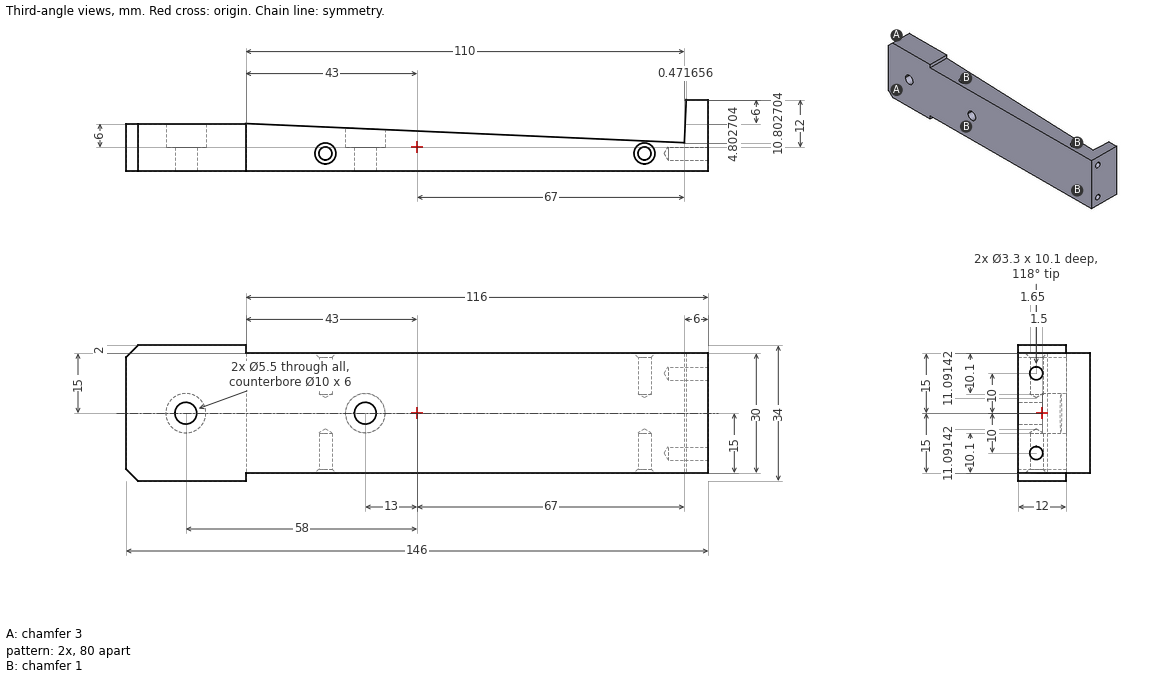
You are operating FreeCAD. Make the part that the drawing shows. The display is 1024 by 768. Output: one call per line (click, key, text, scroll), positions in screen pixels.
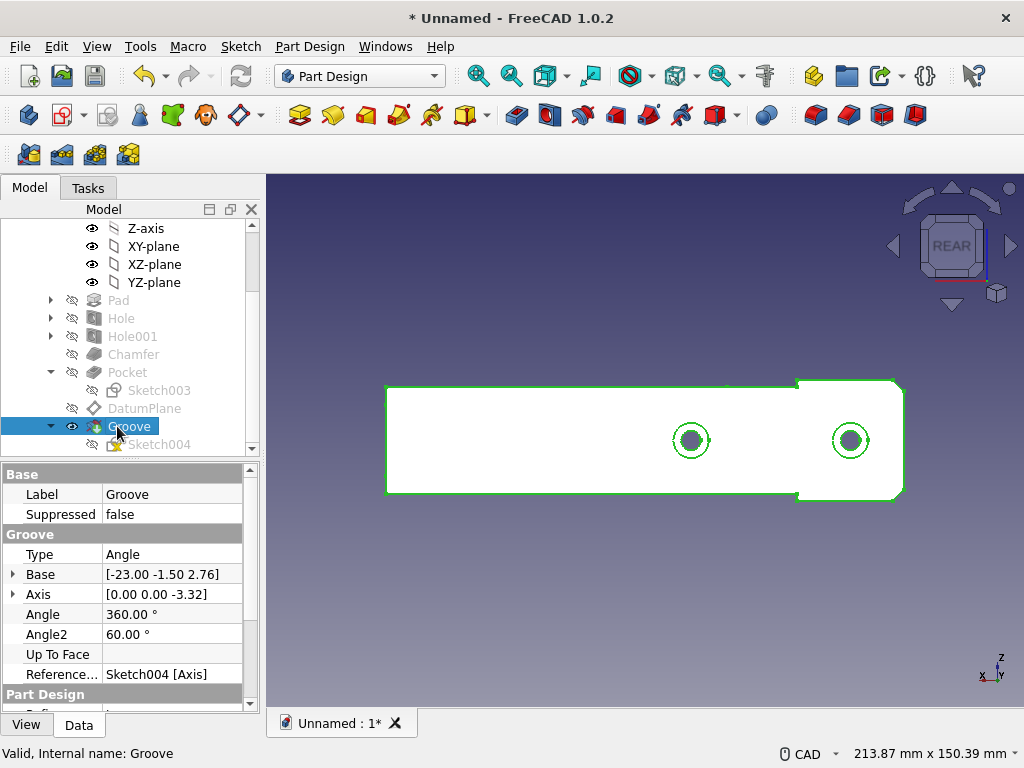
click(62, 154)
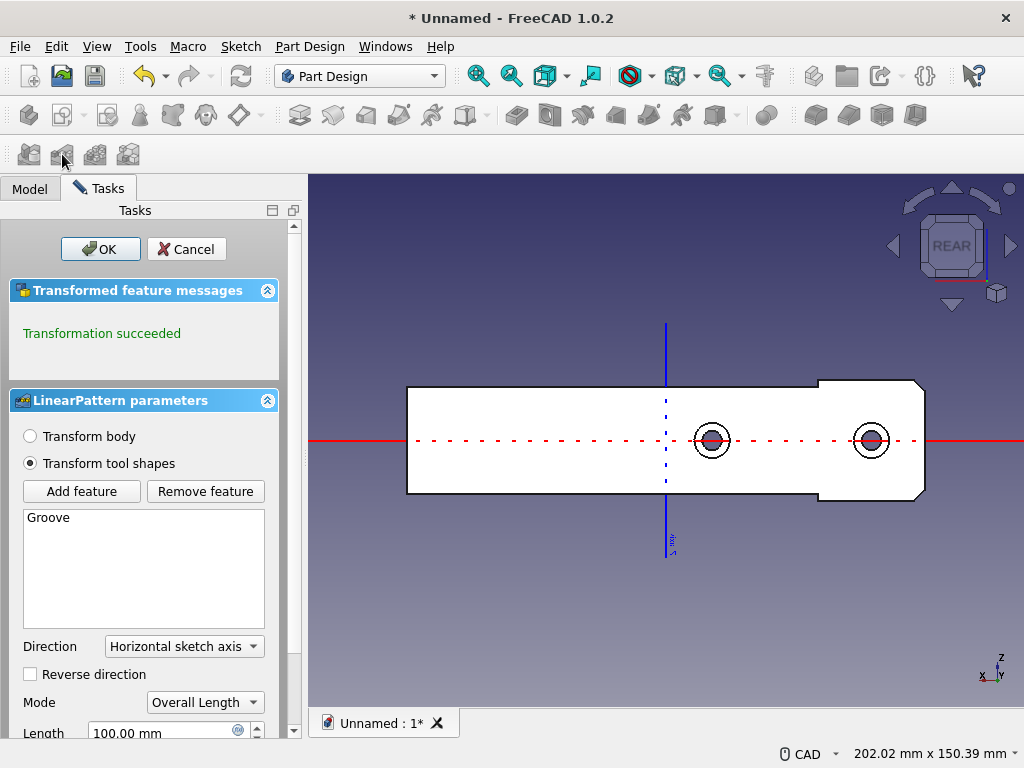
click(185, 646)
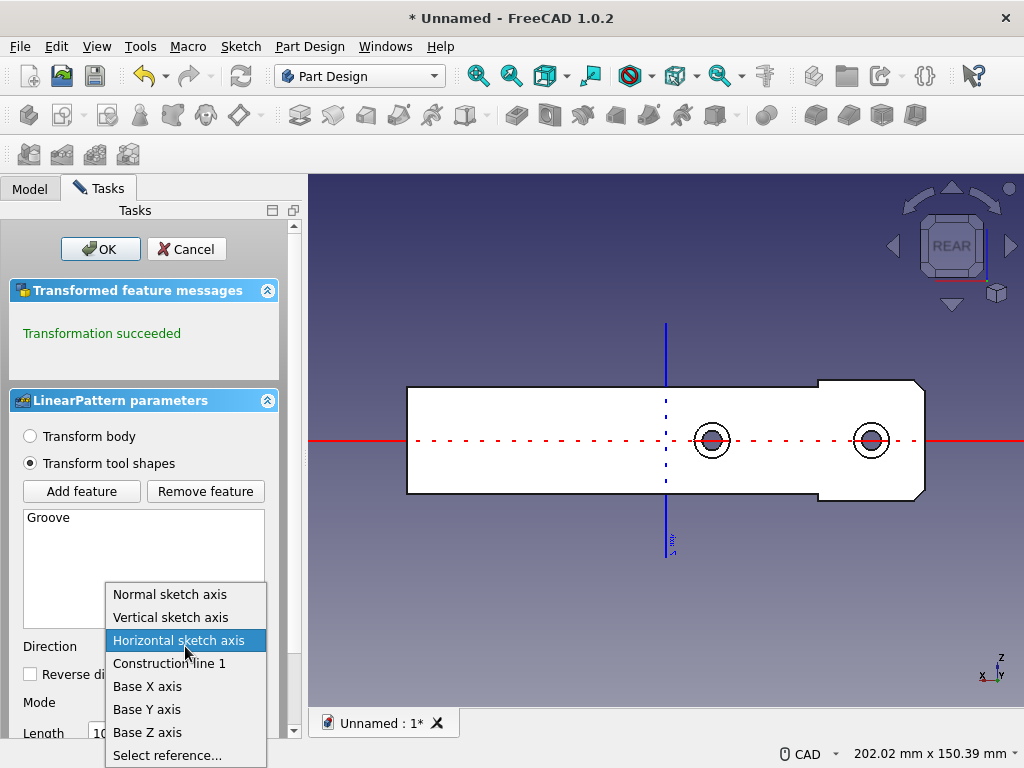
click(184, 686)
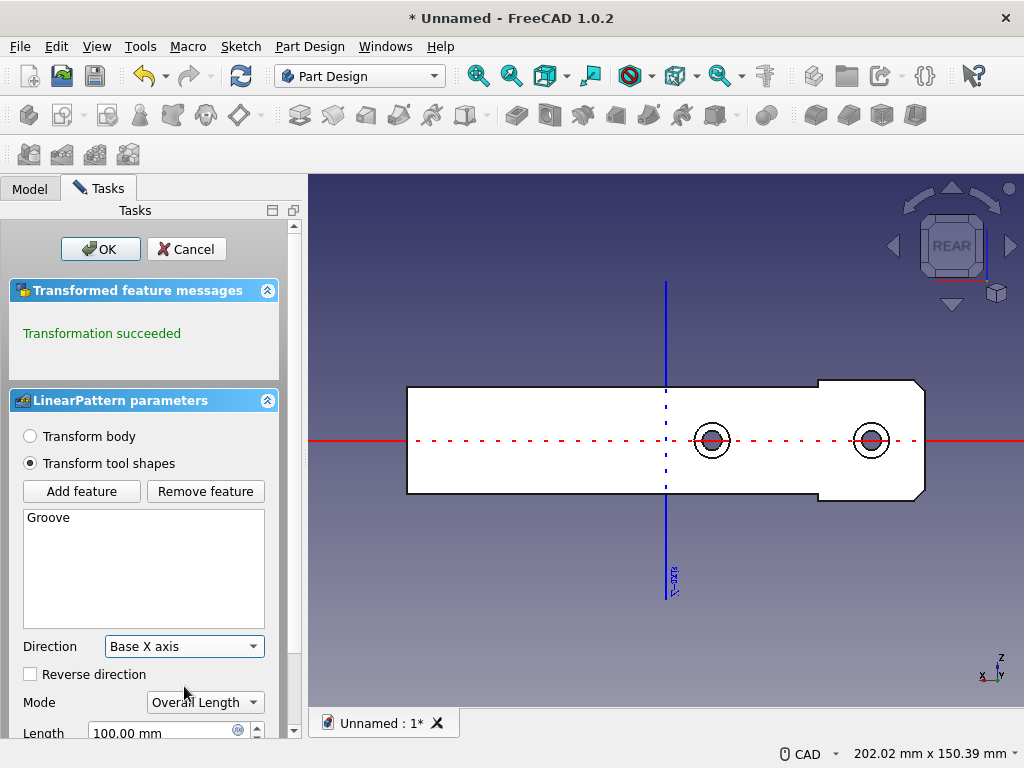
click(206, 702)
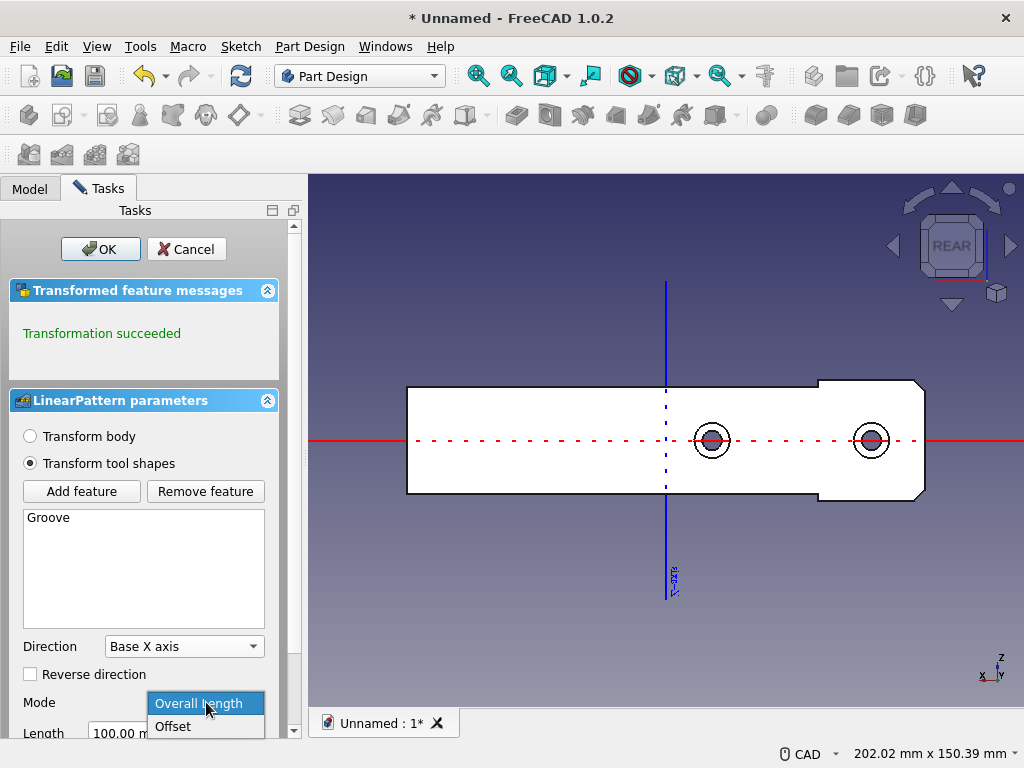
click(204, 726)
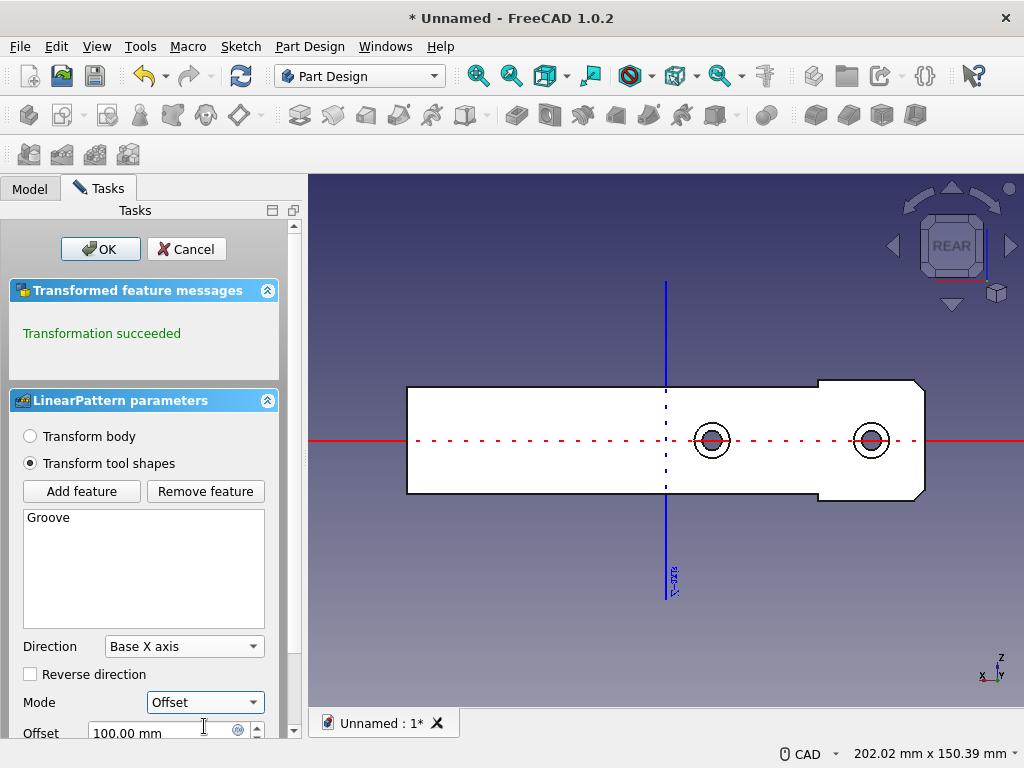
scroll(294, 479, down, 2)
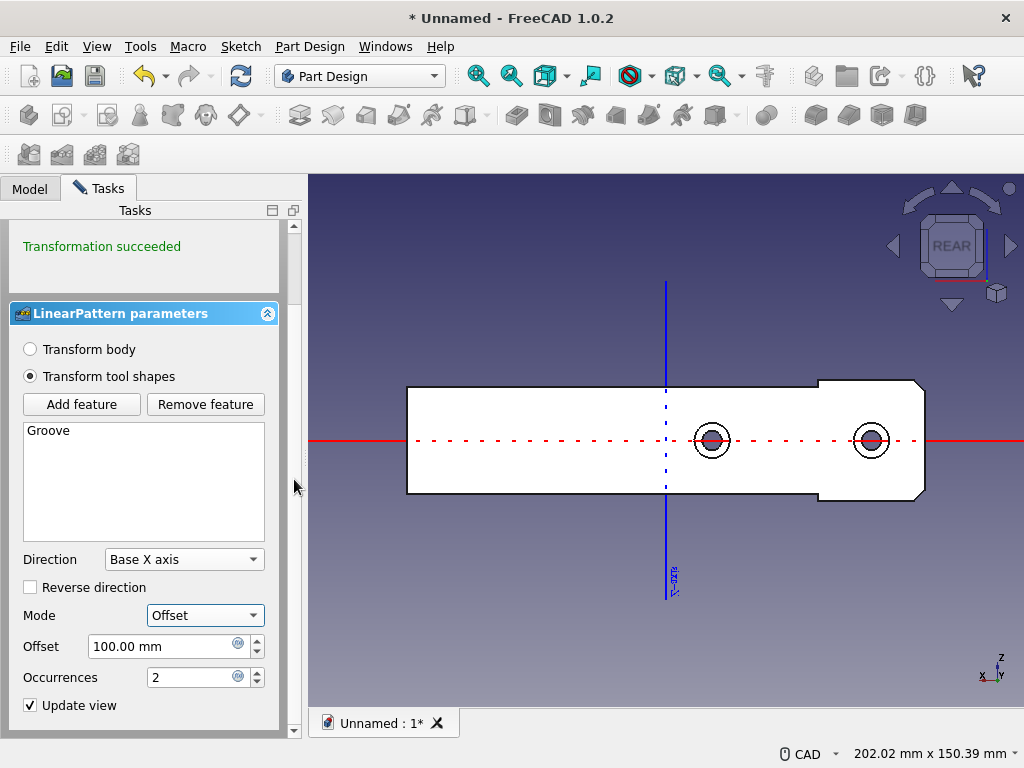
triple_click(170, 646)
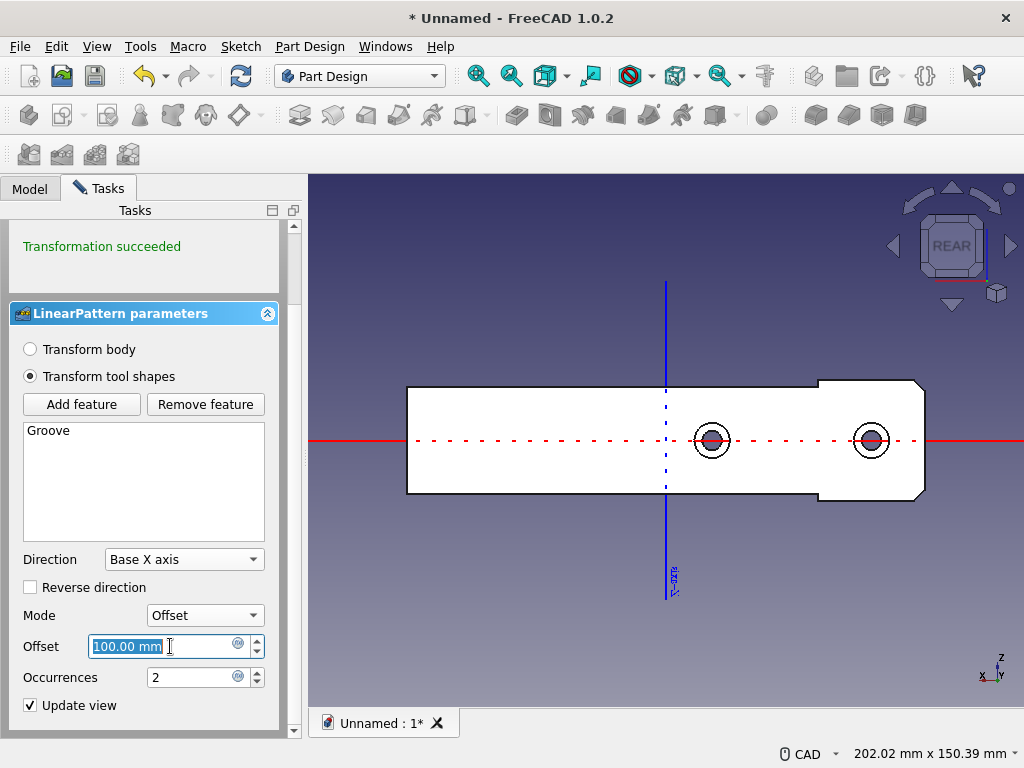
text(80)
key(Tab)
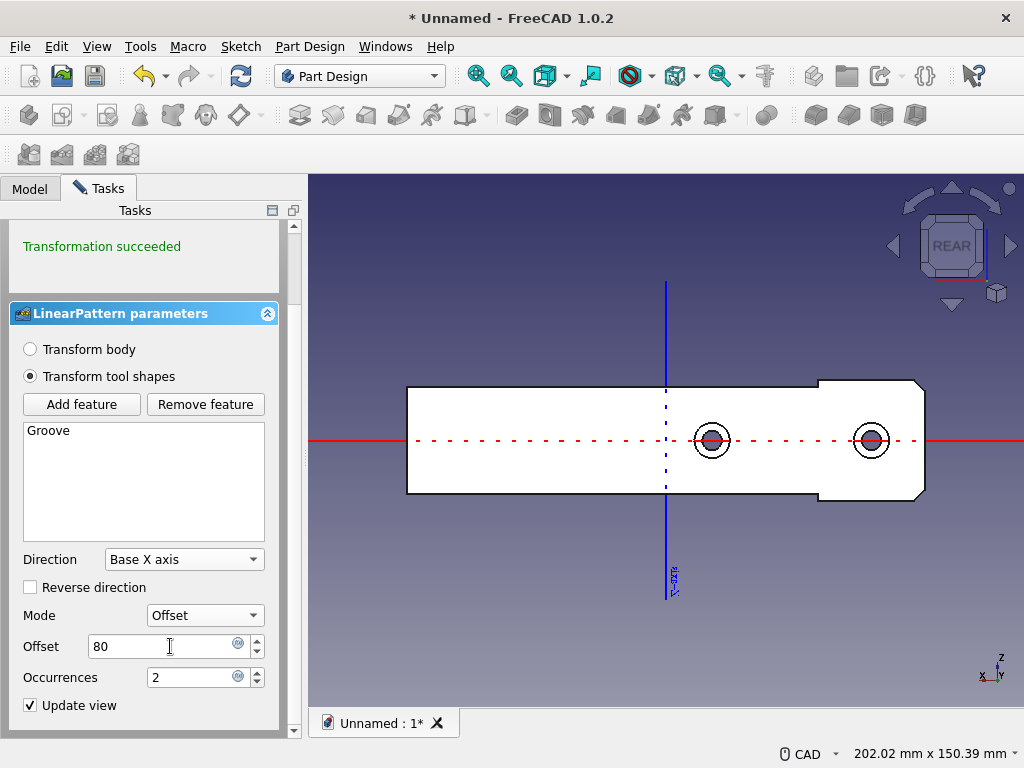
triple_click(199, 678)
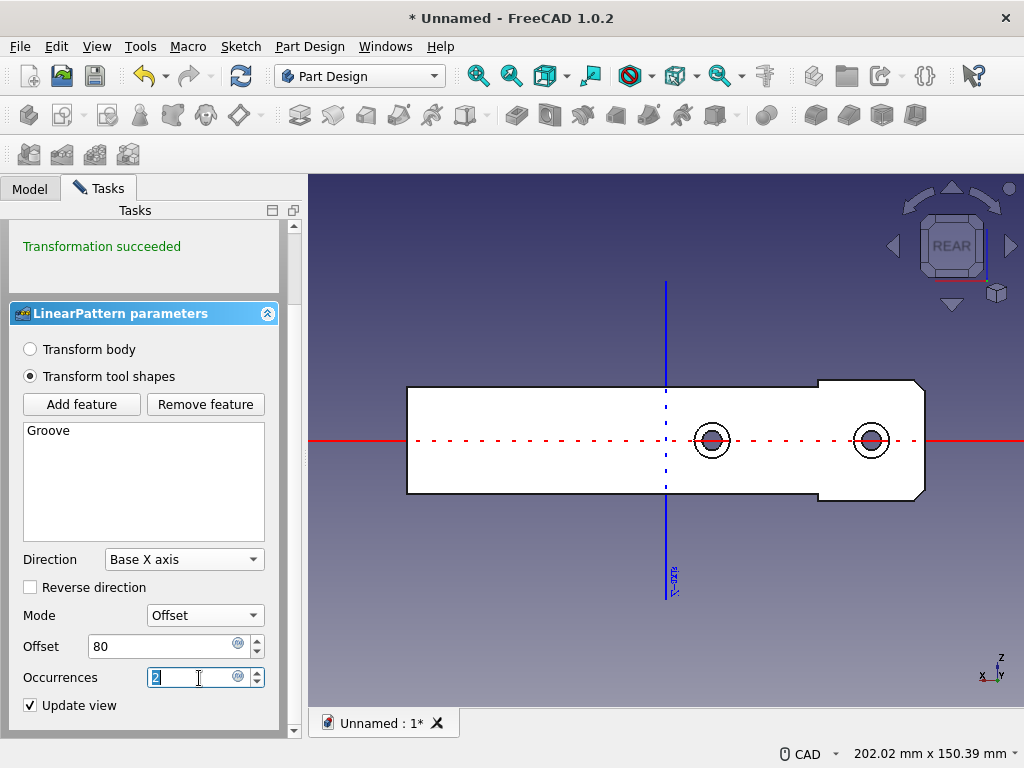
text(2)
key(Tab)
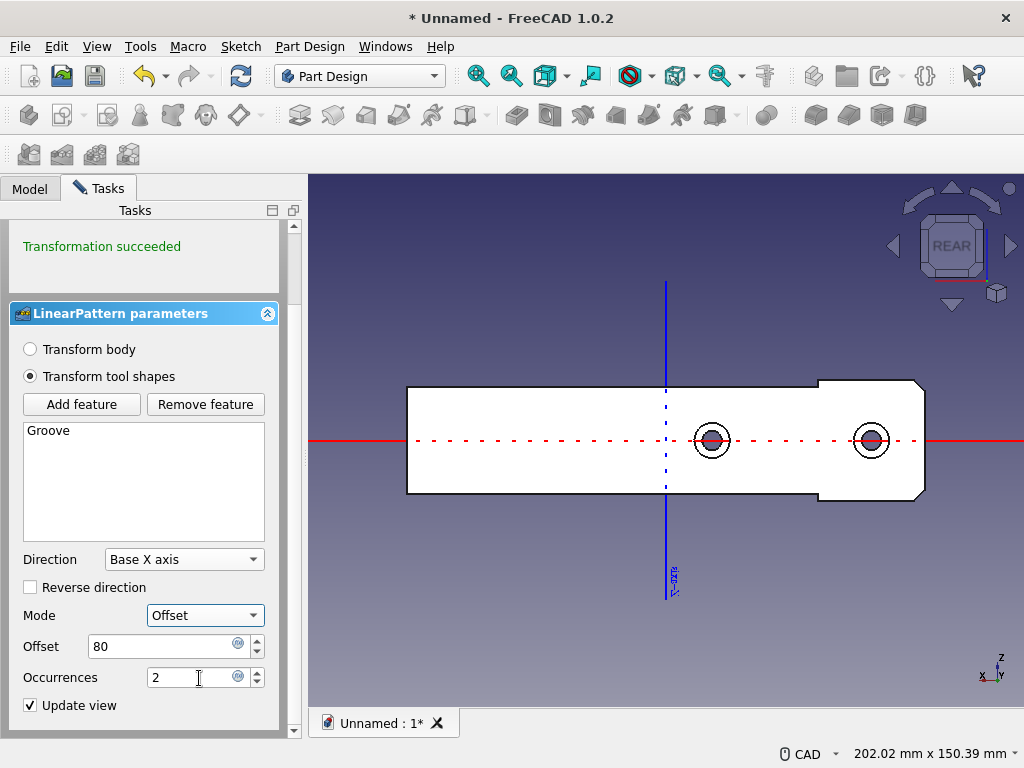
scroll(294, 479, up, 3)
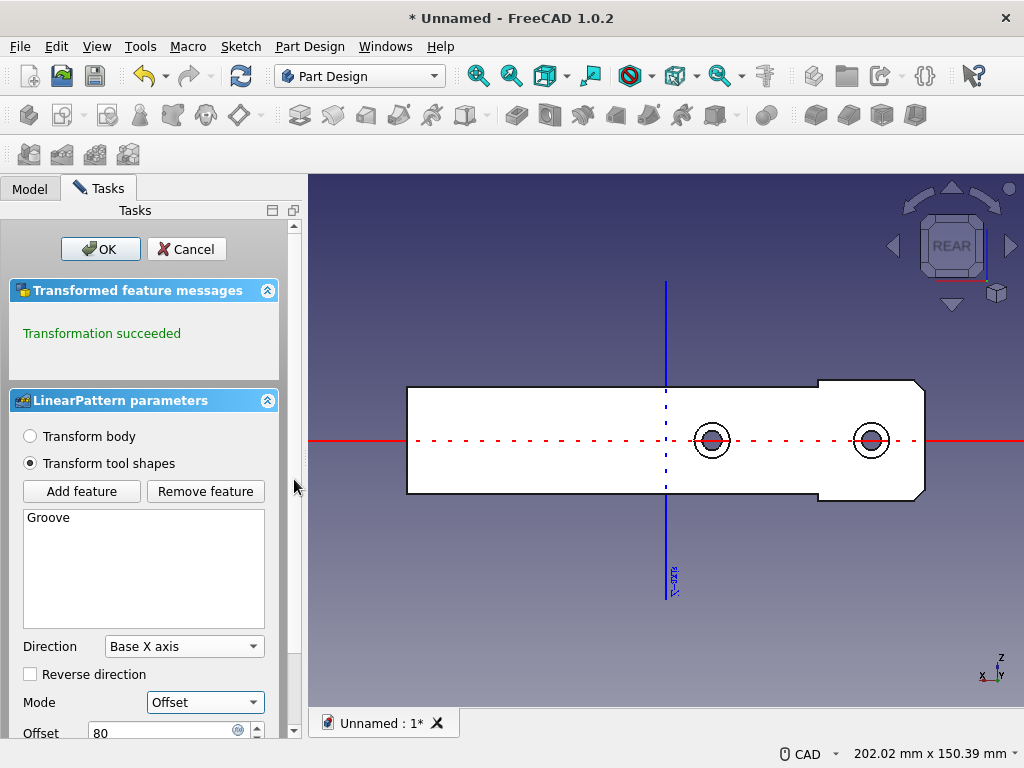
click(101, 249)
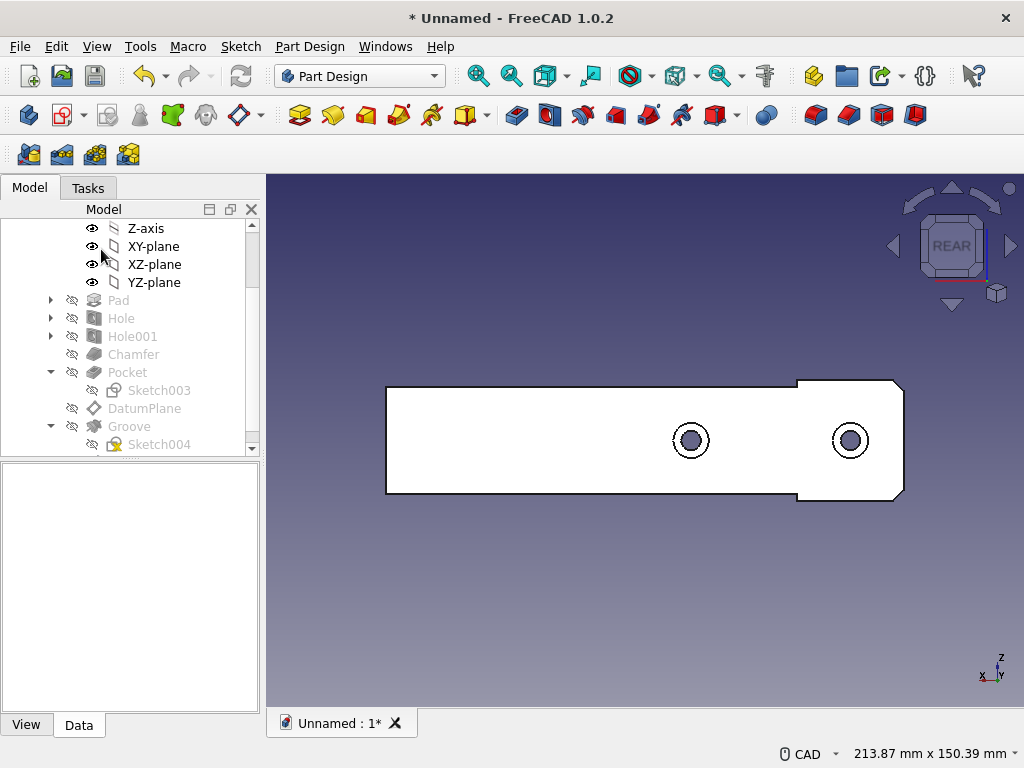
click(117, 426)